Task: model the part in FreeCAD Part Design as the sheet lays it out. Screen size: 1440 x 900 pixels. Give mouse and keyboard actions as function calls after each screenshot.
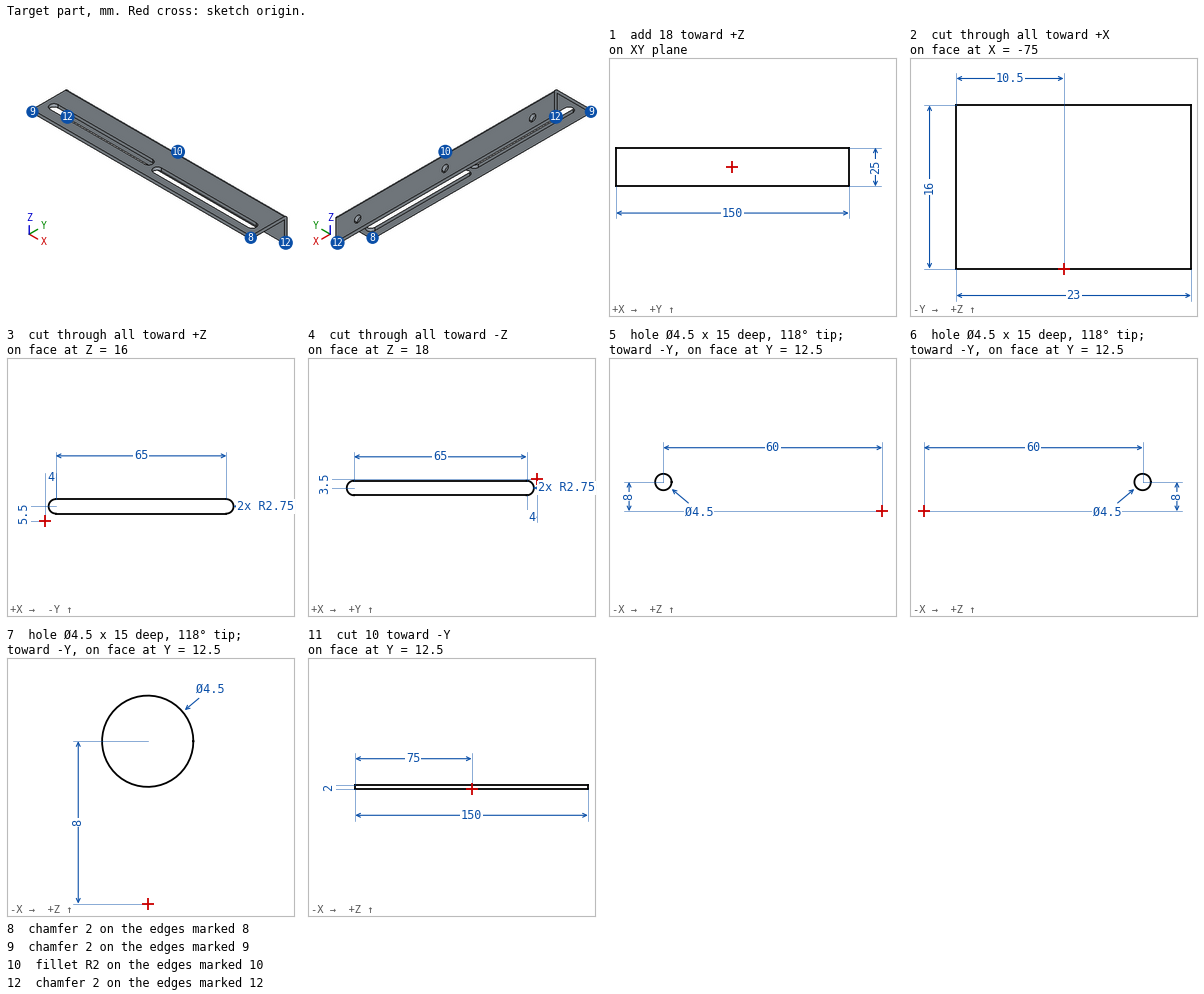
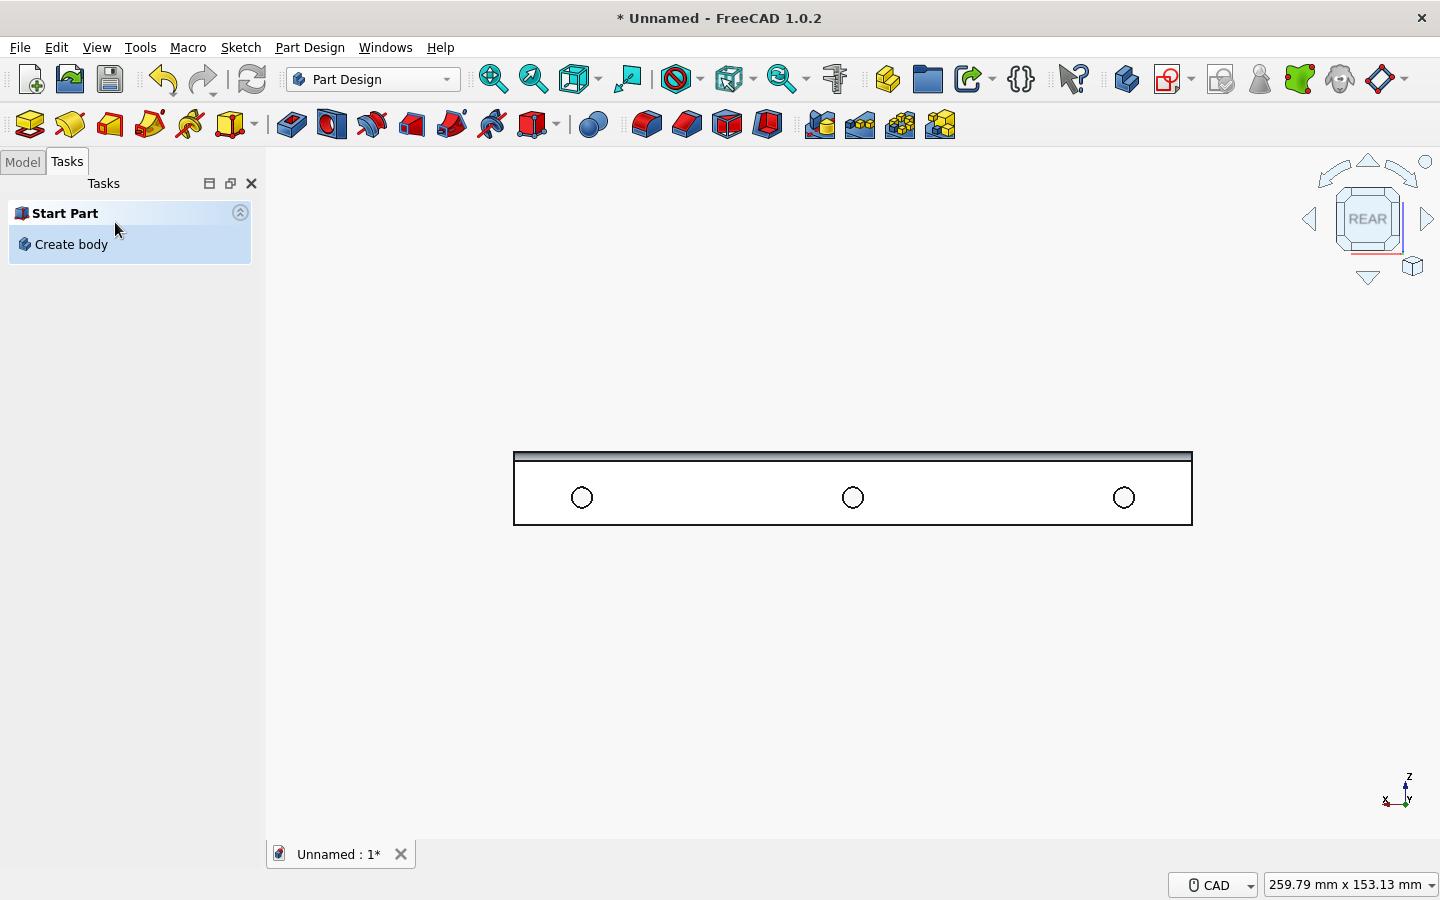
scroll(514, 524, up, 8)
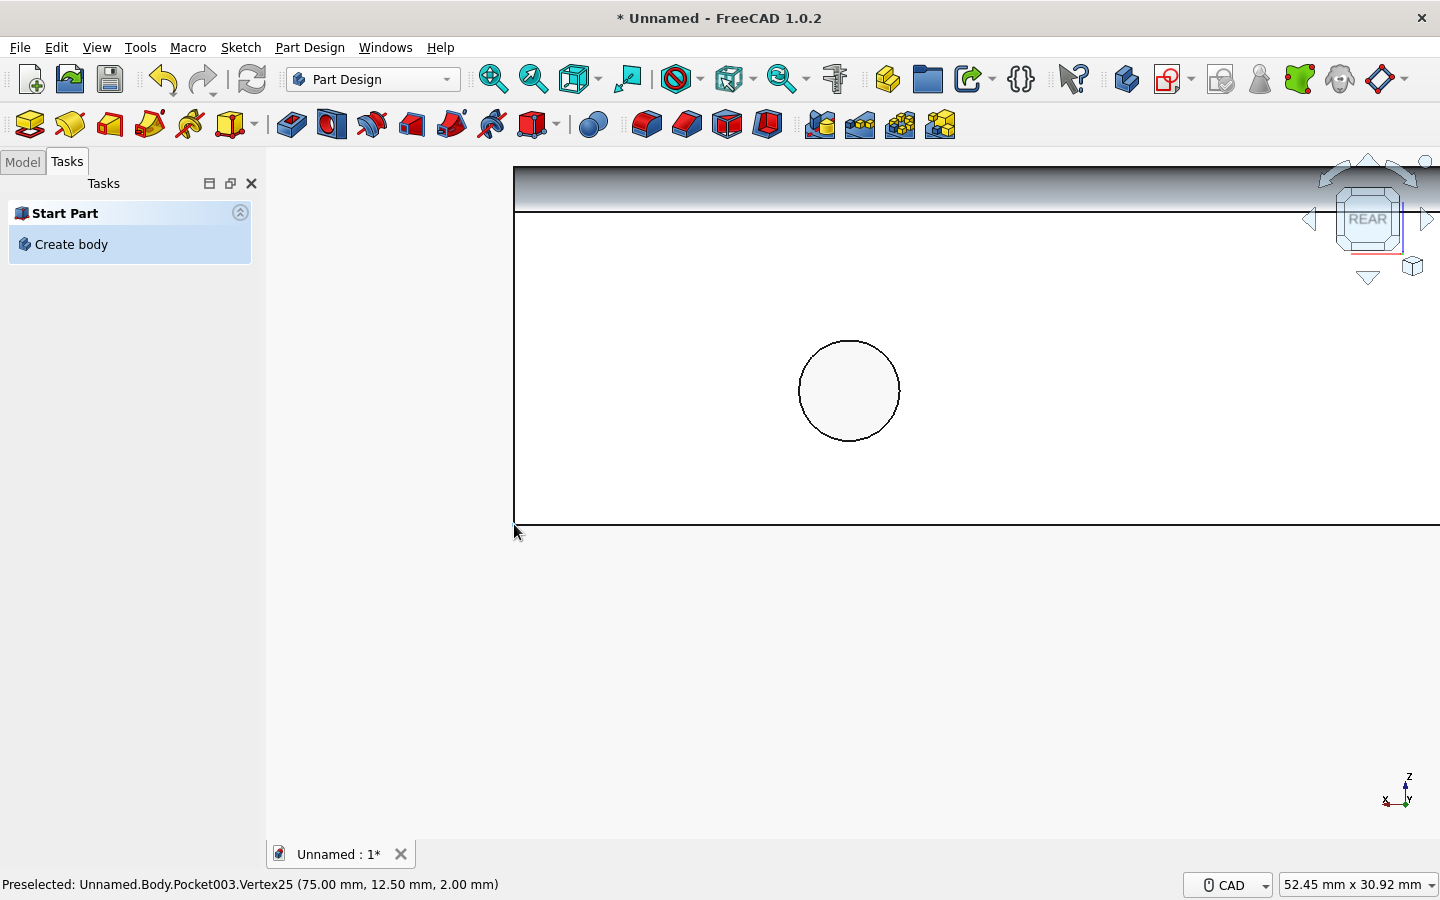
click(494, 80)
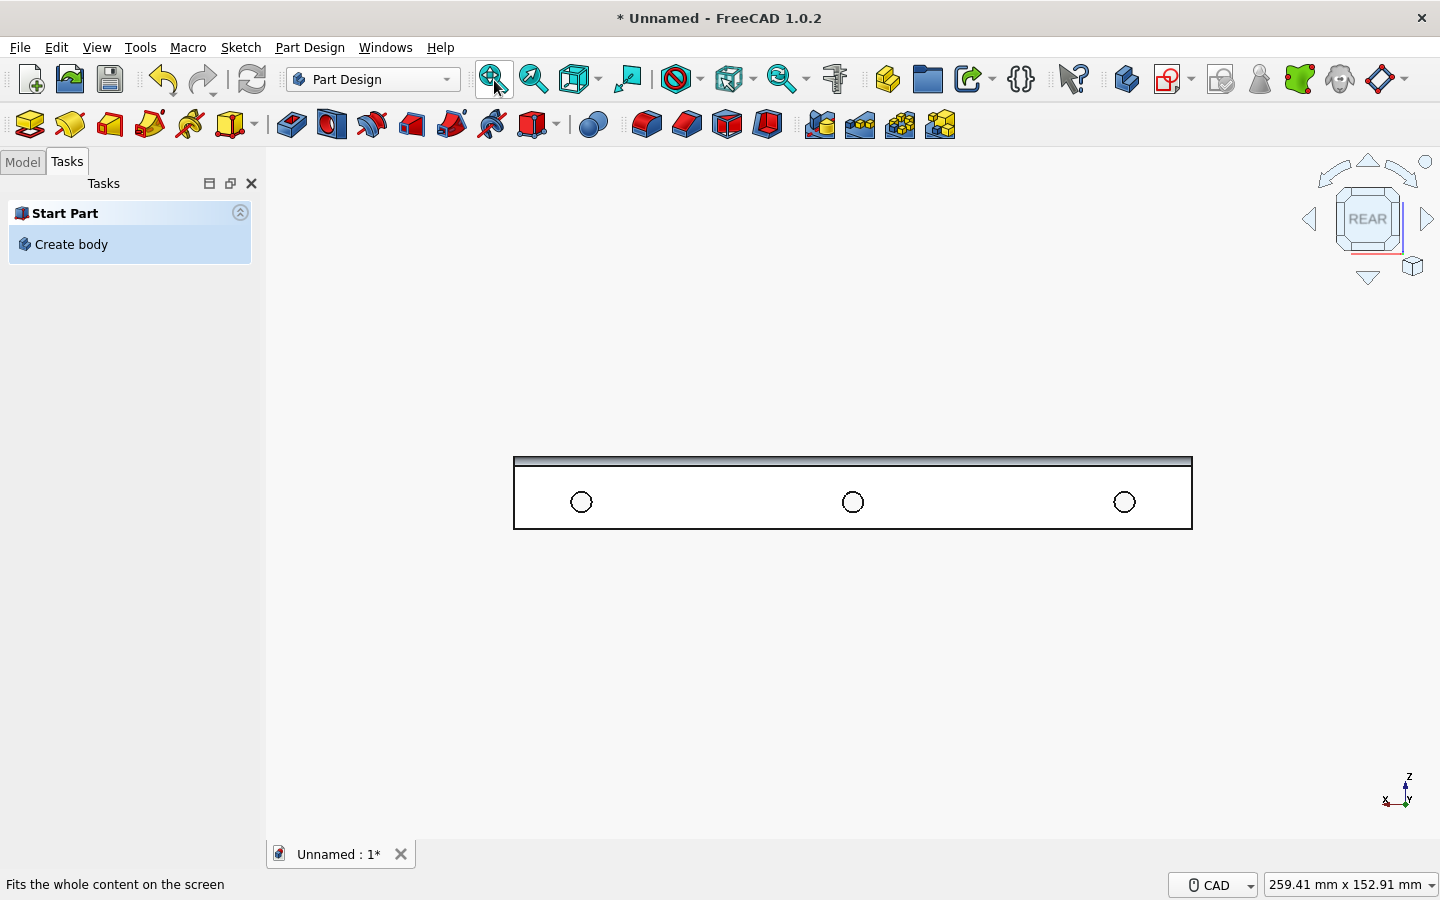
key(0)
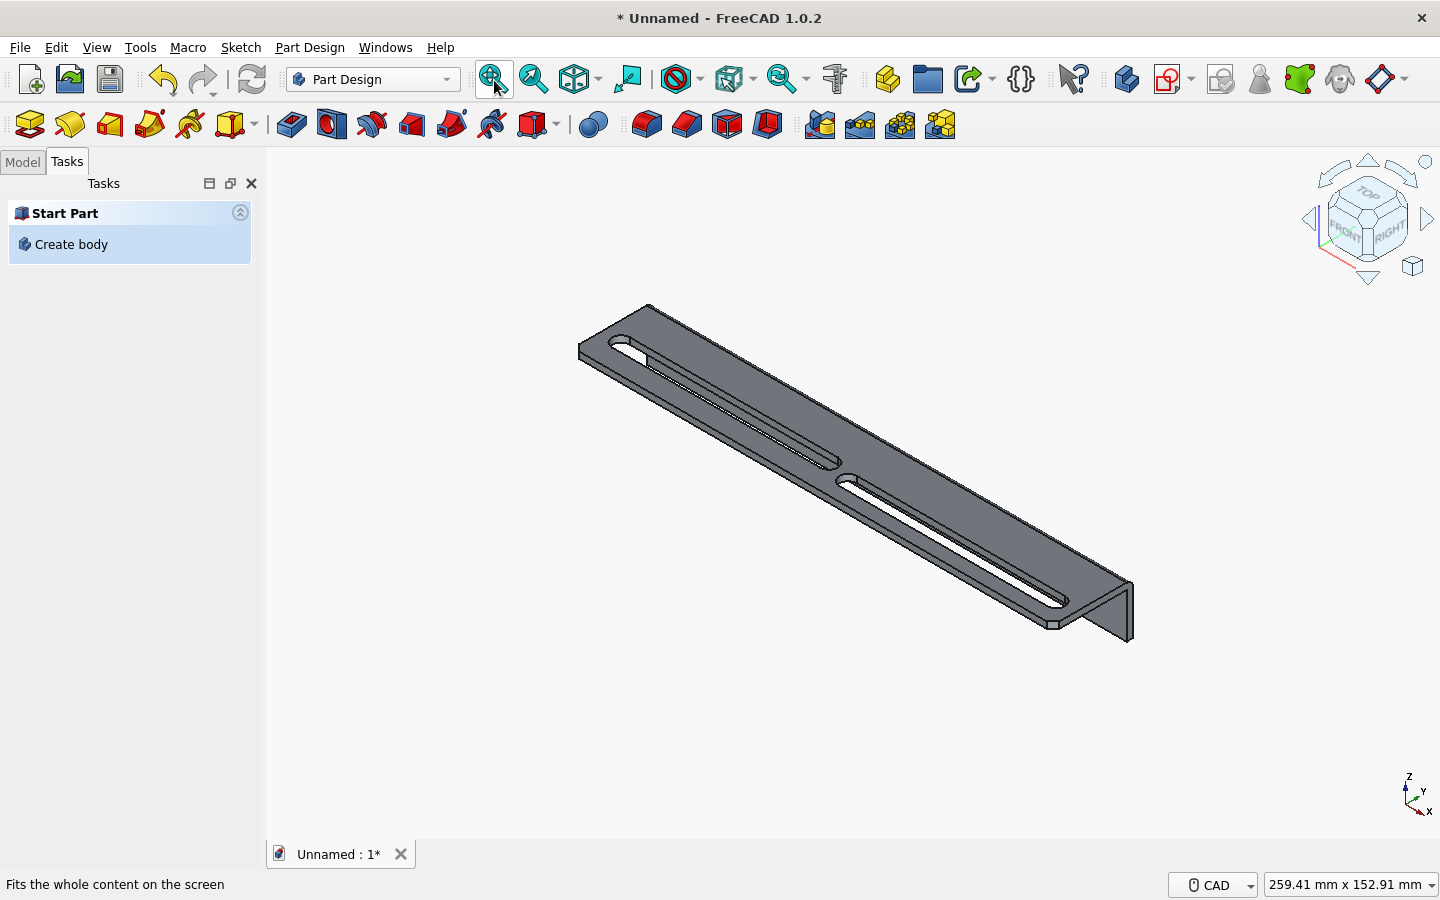
scroll(1130, 639, up, 8)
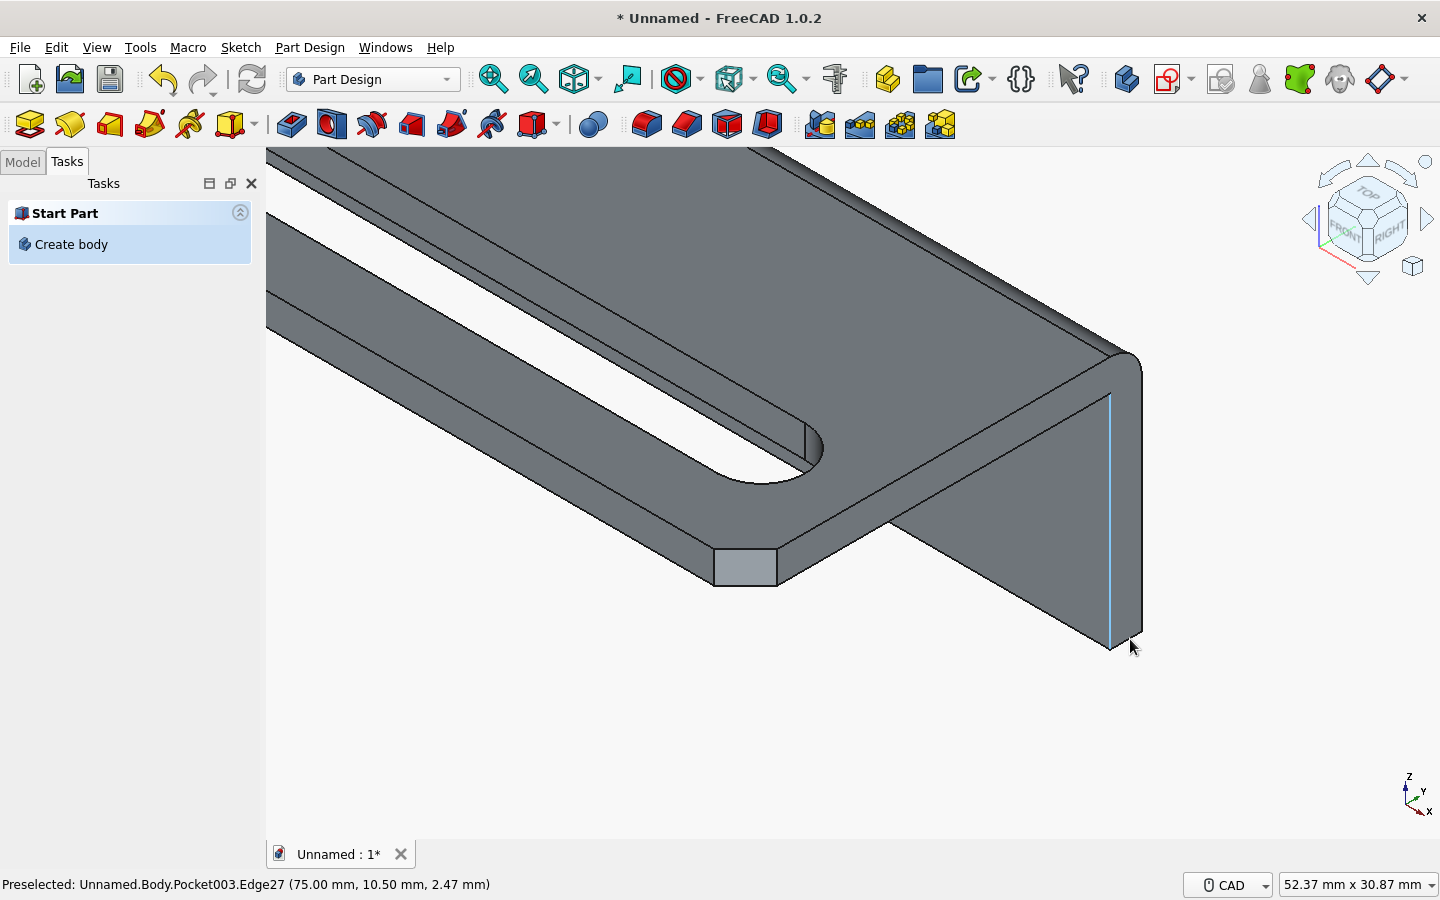
click(494, 80)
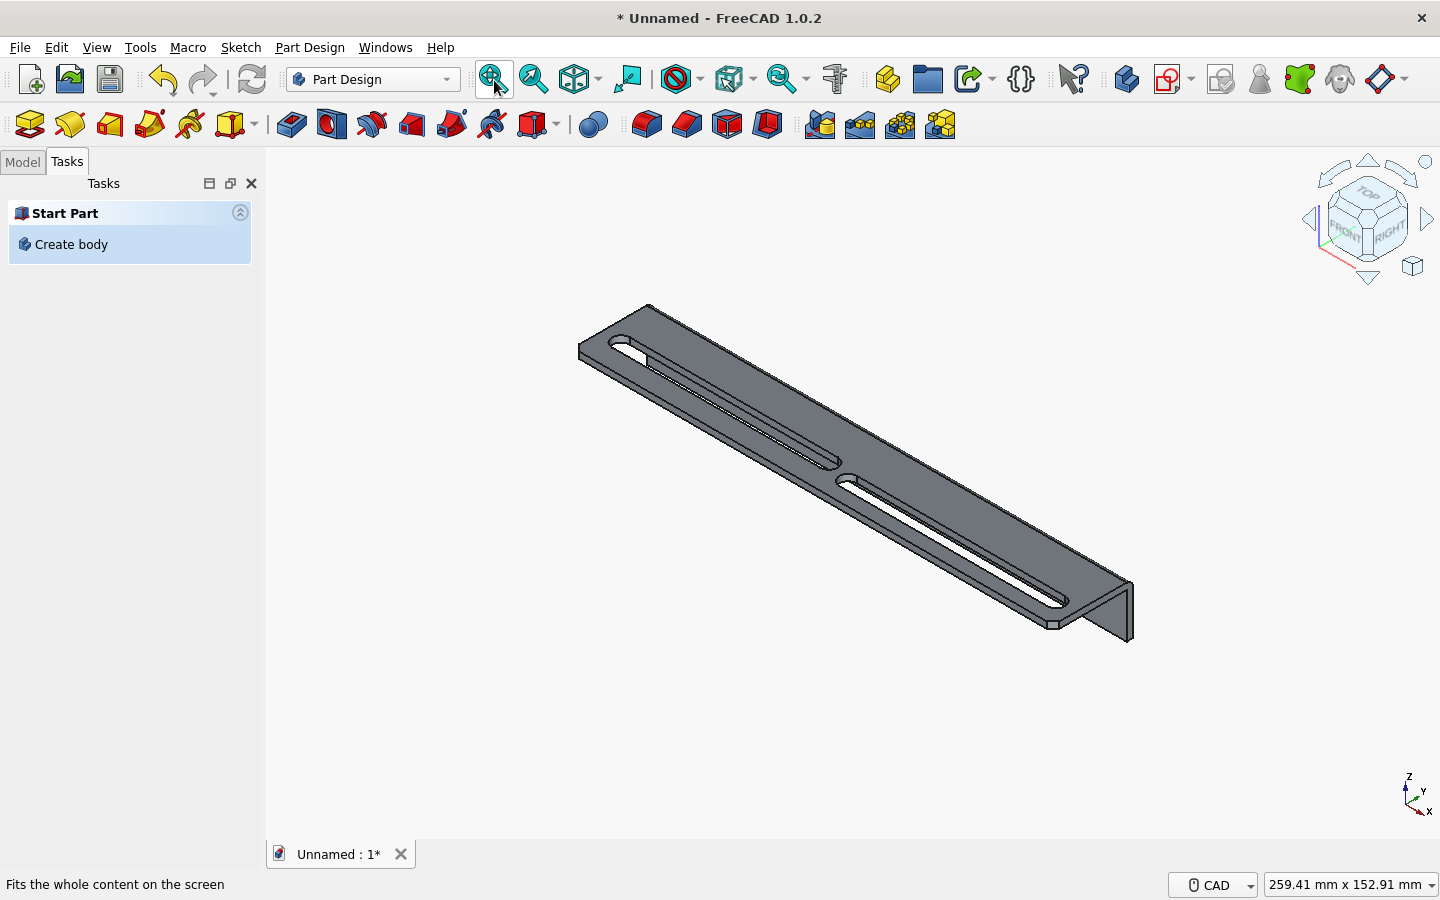
key(2)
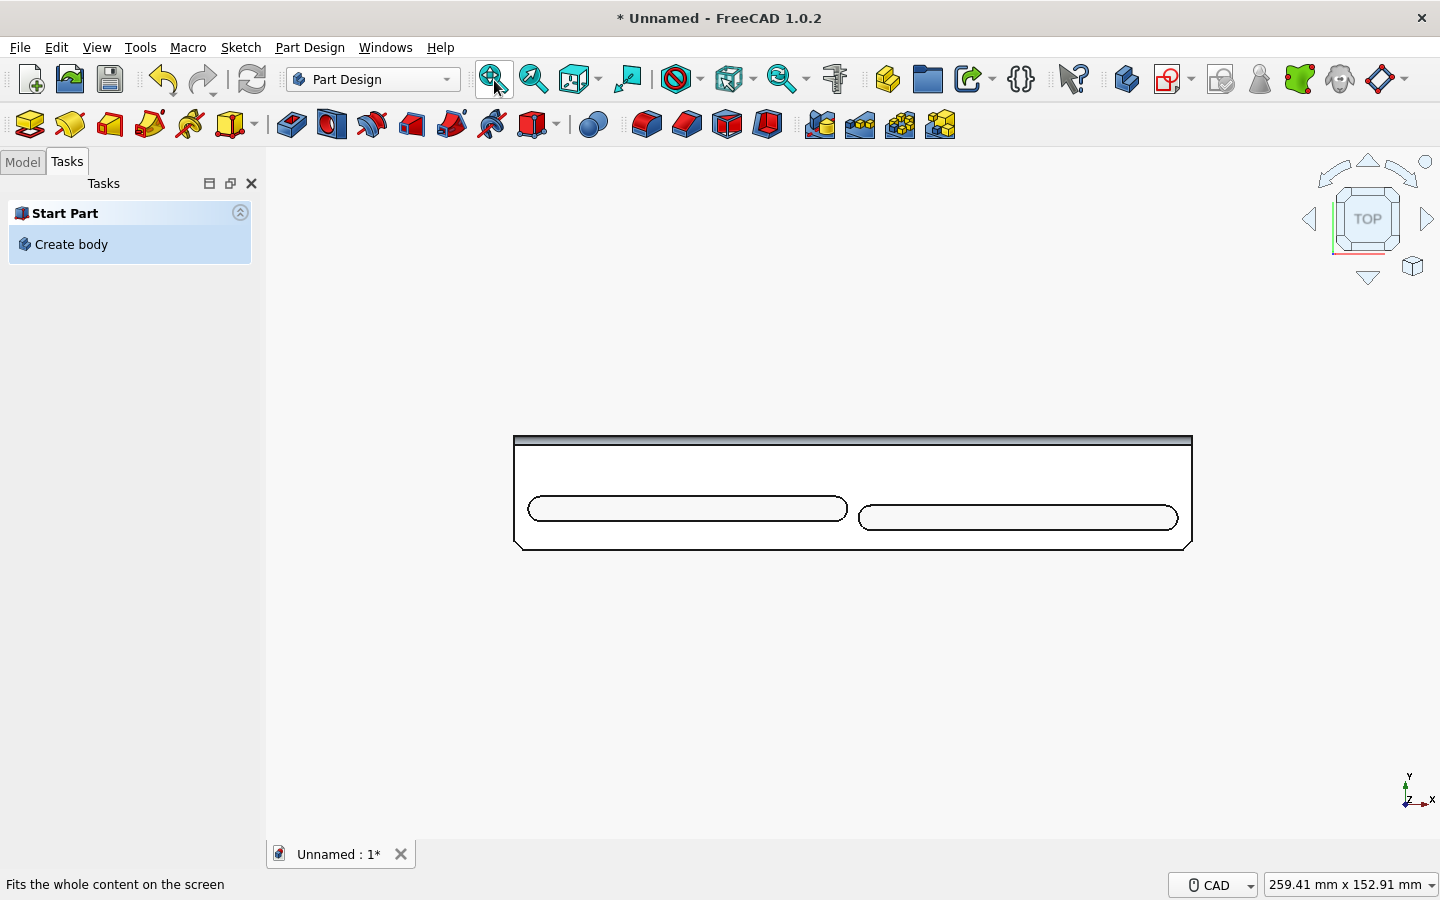
scroll(1192, 440, up, 8)